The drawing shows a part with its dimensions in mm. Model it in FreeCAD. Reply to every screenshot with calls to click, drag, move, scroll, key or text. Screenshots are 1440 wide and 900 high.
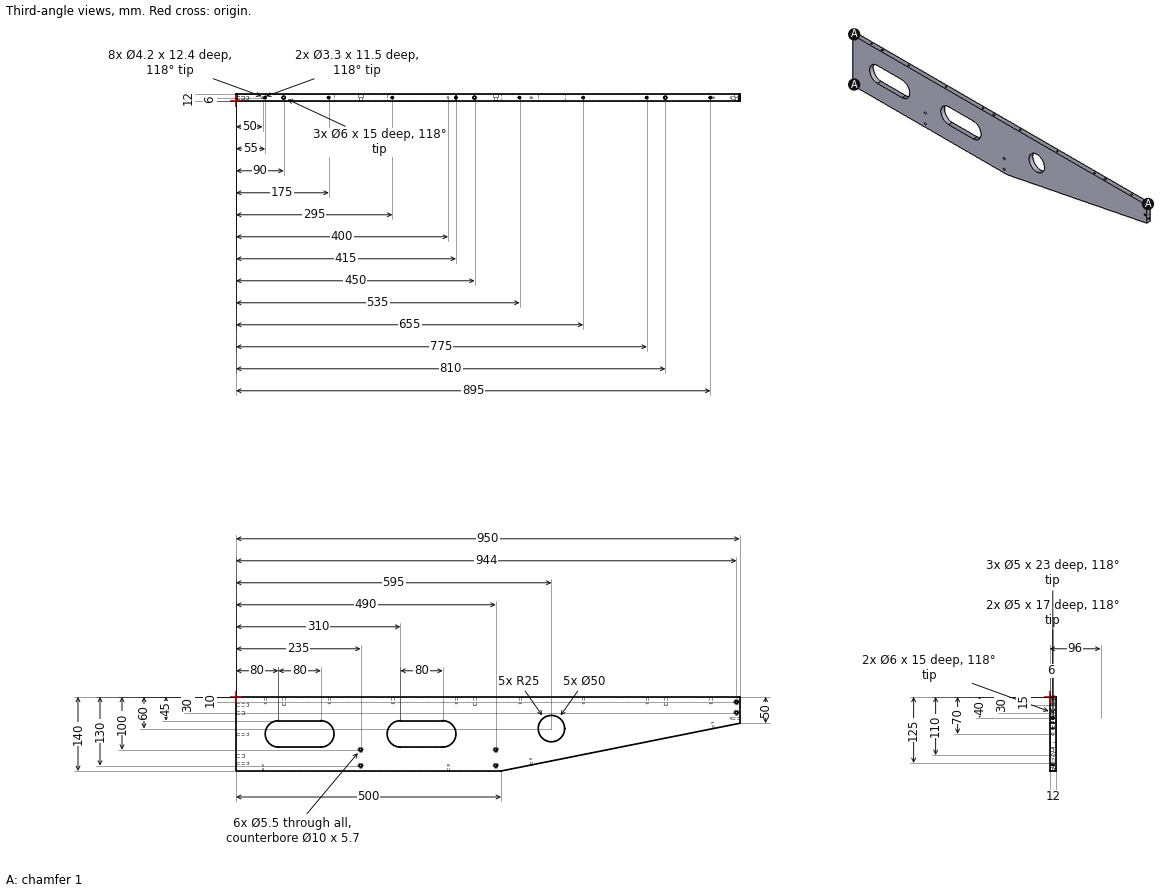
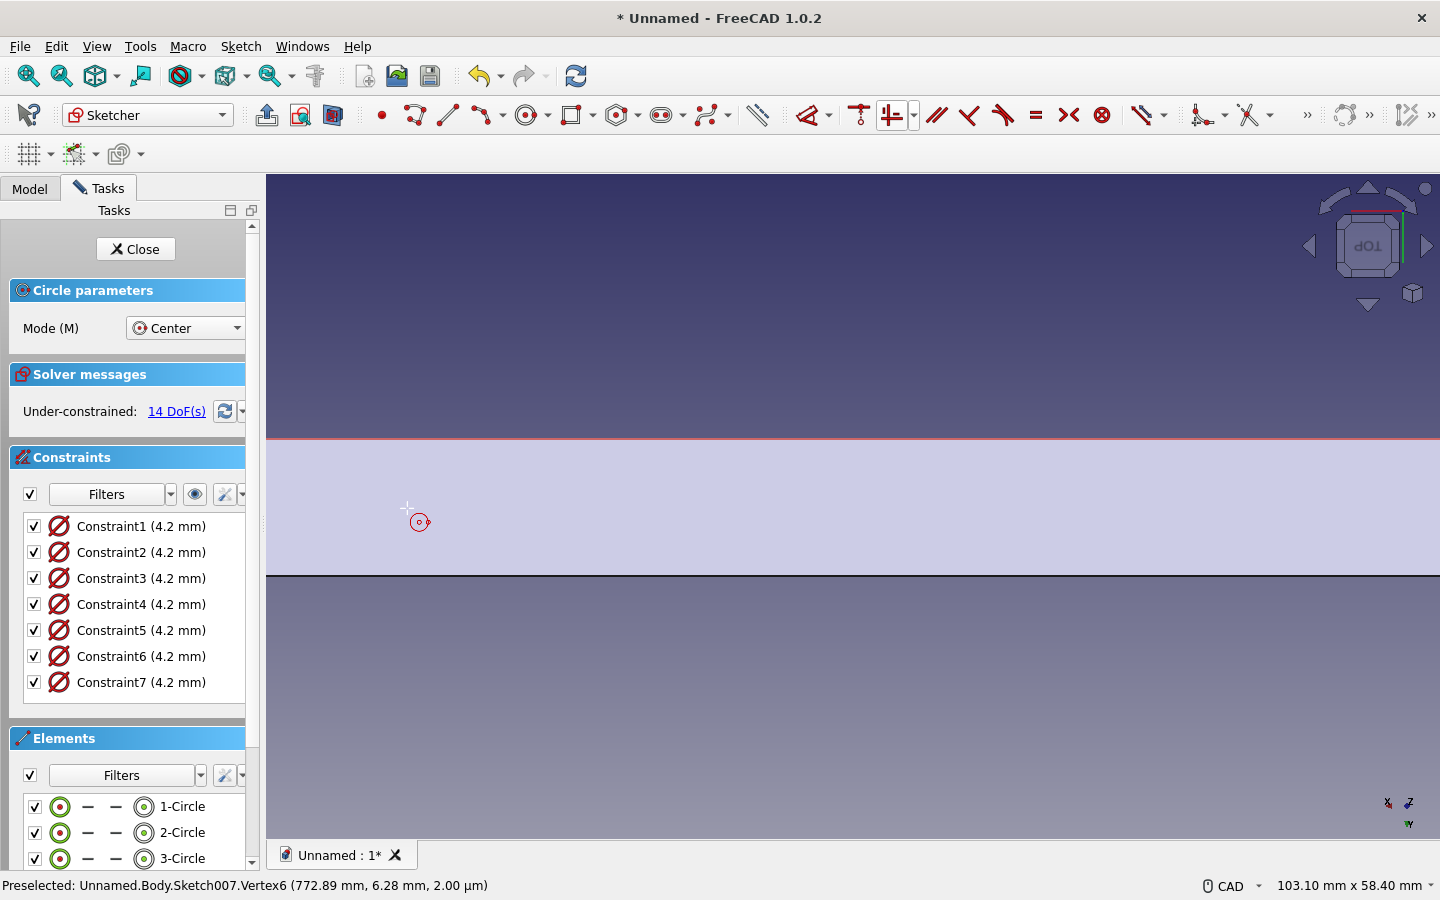
scroll(407, 508, down, 13)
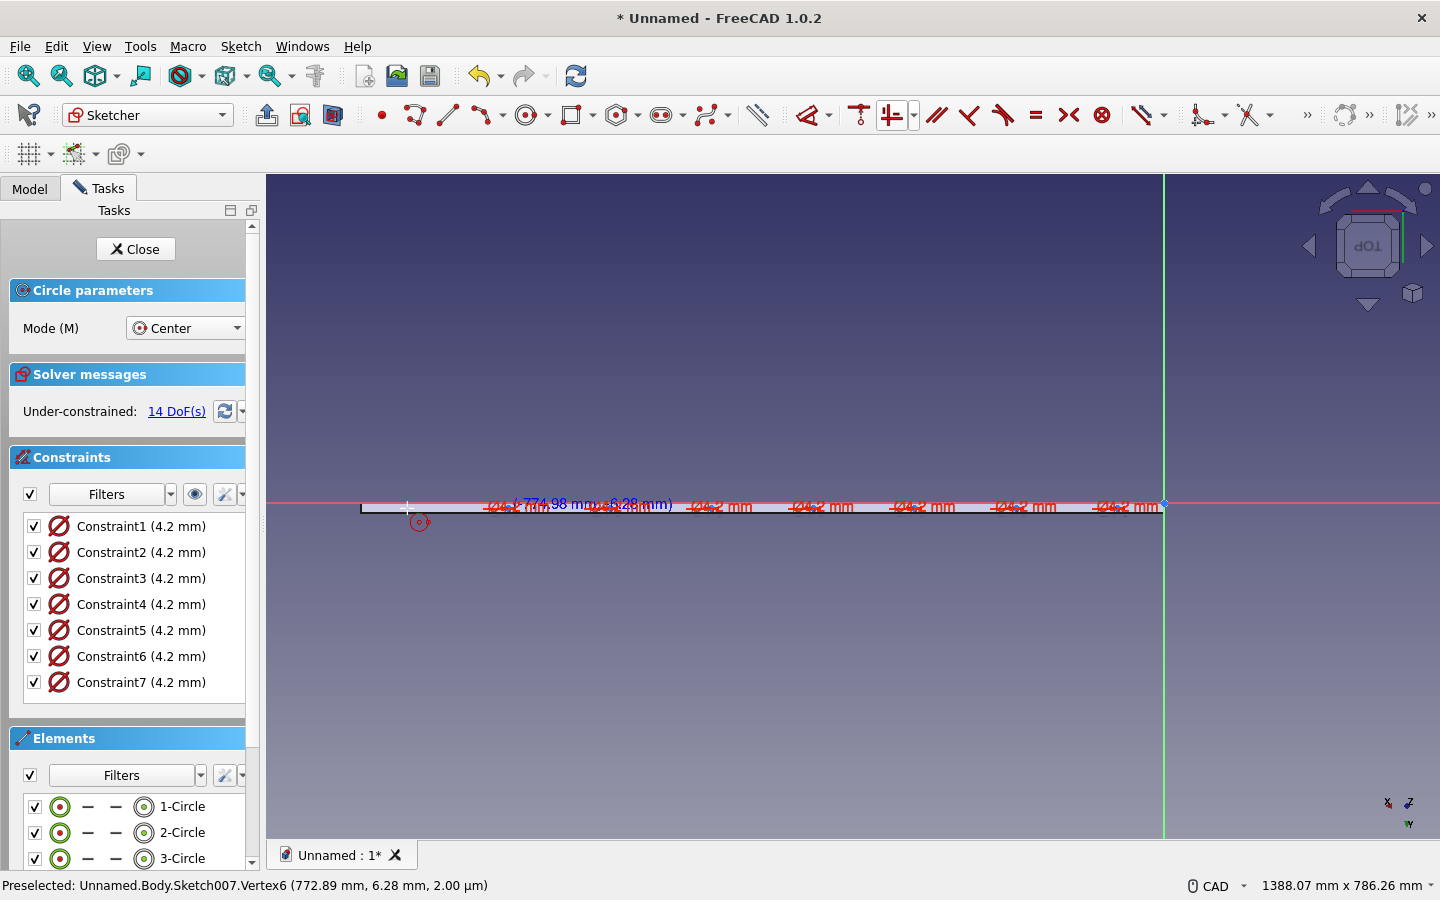
scroll(407, 508, up, 6)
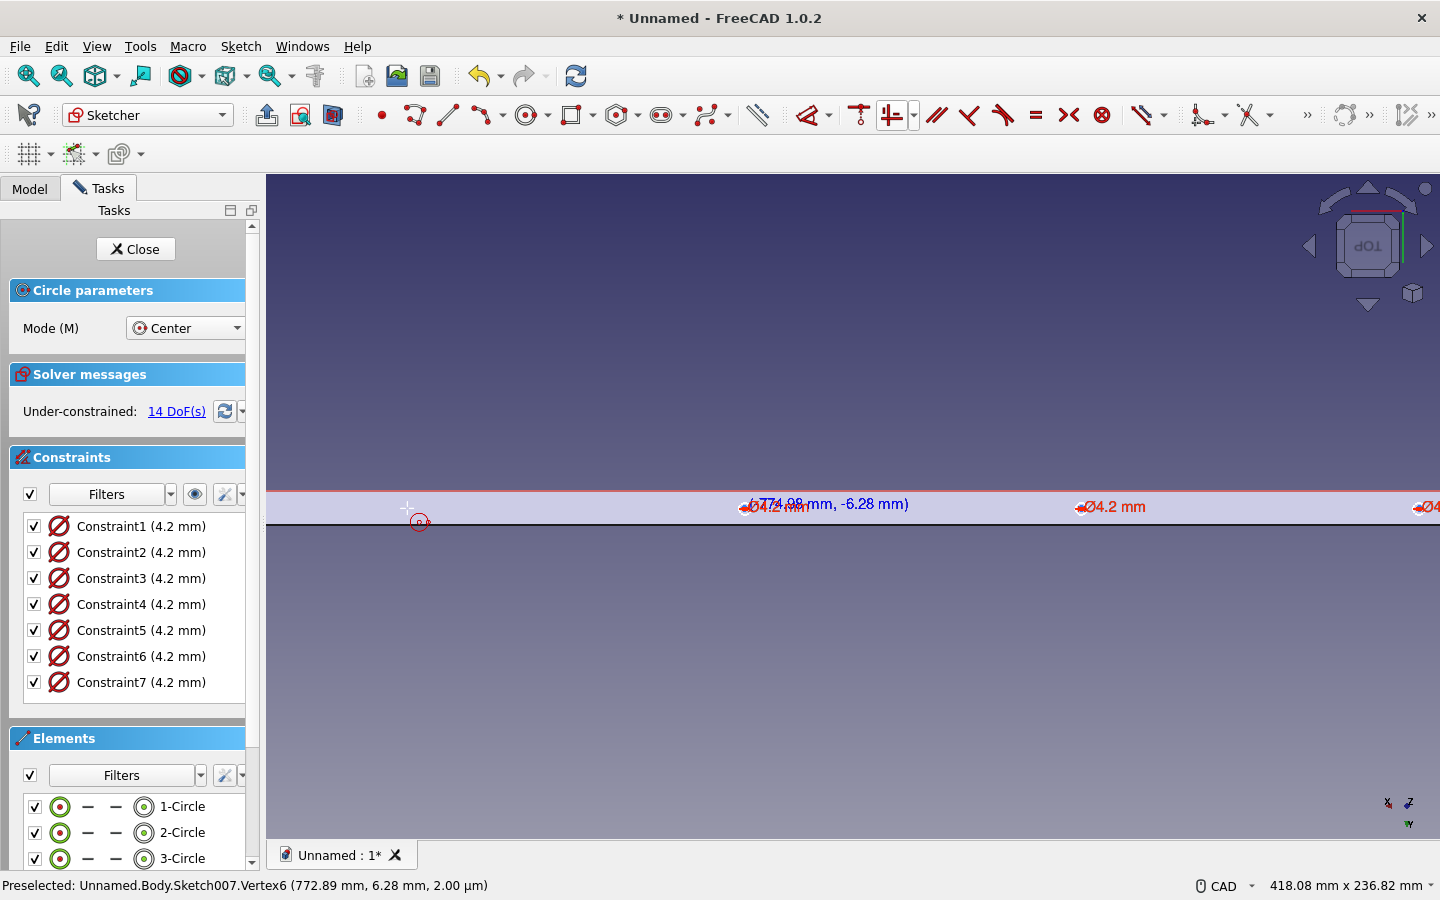
click(408, 508)
move(412, 512)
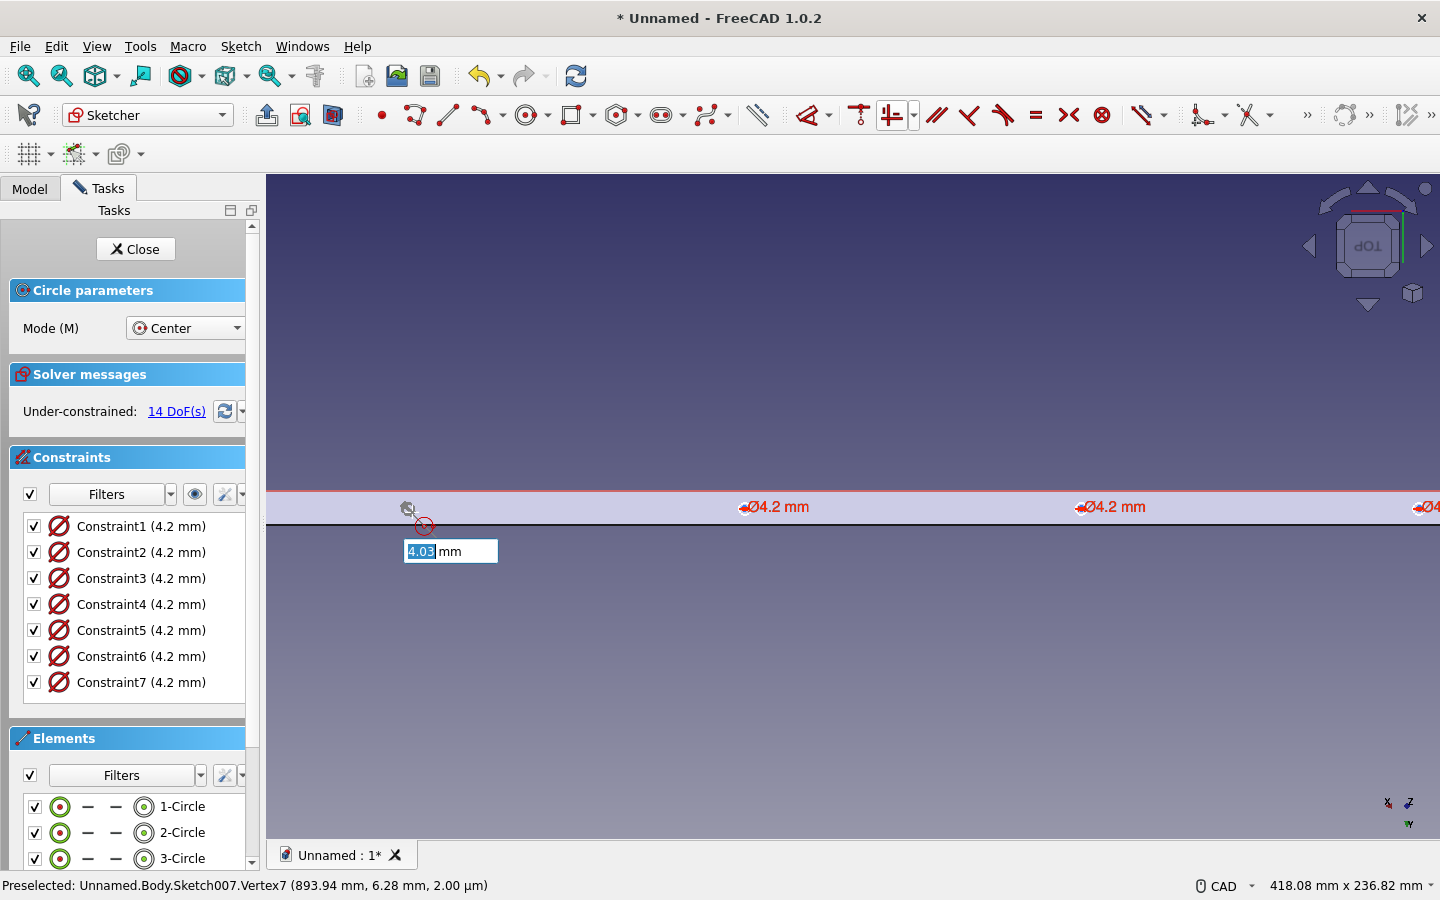
text(4.2)
key(Return)
key(Escape)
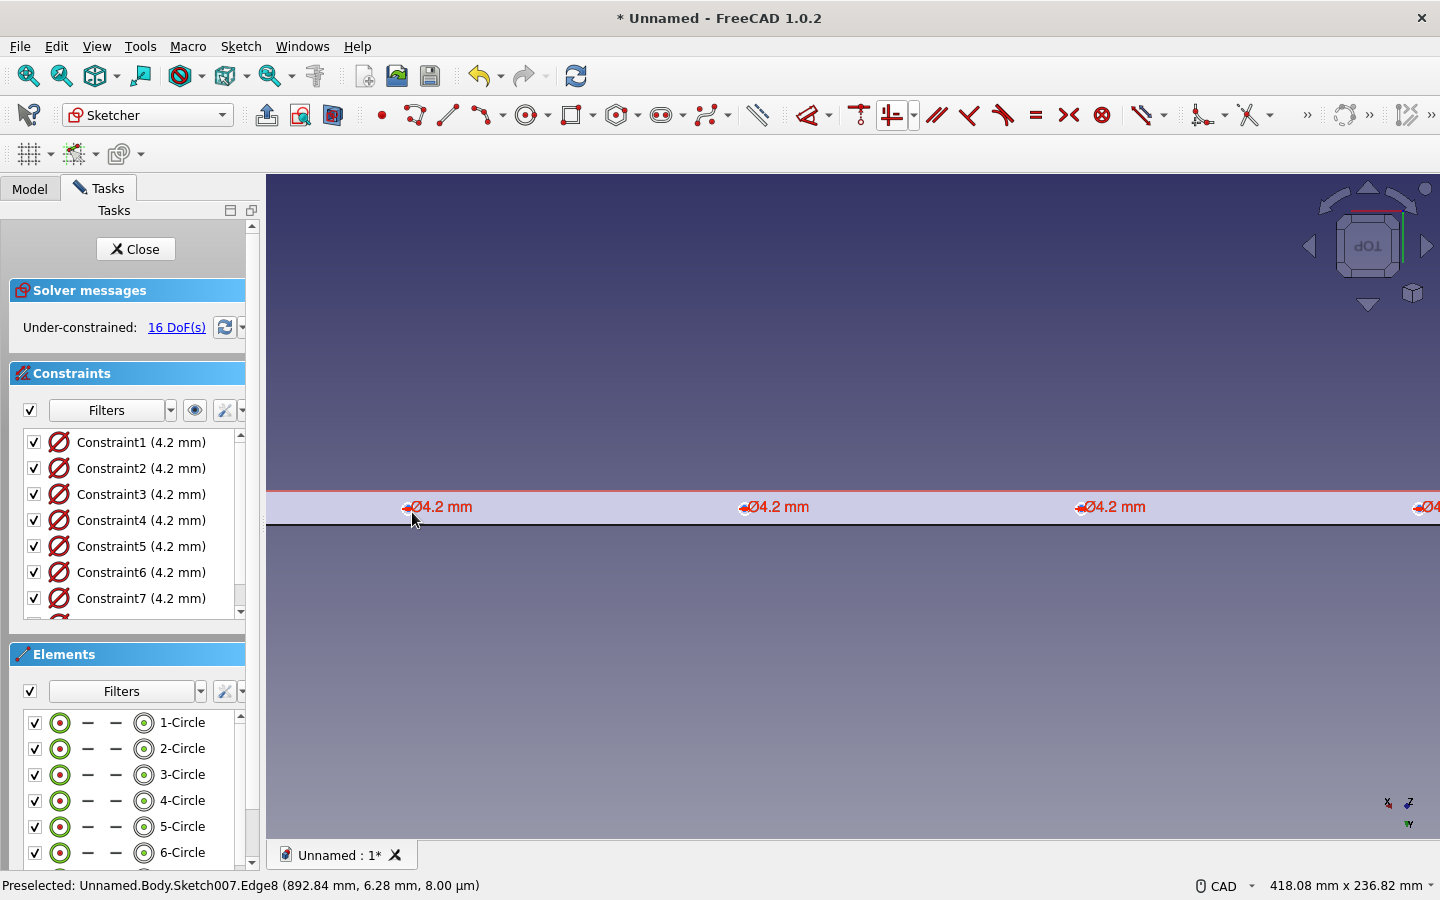
click(806, 116)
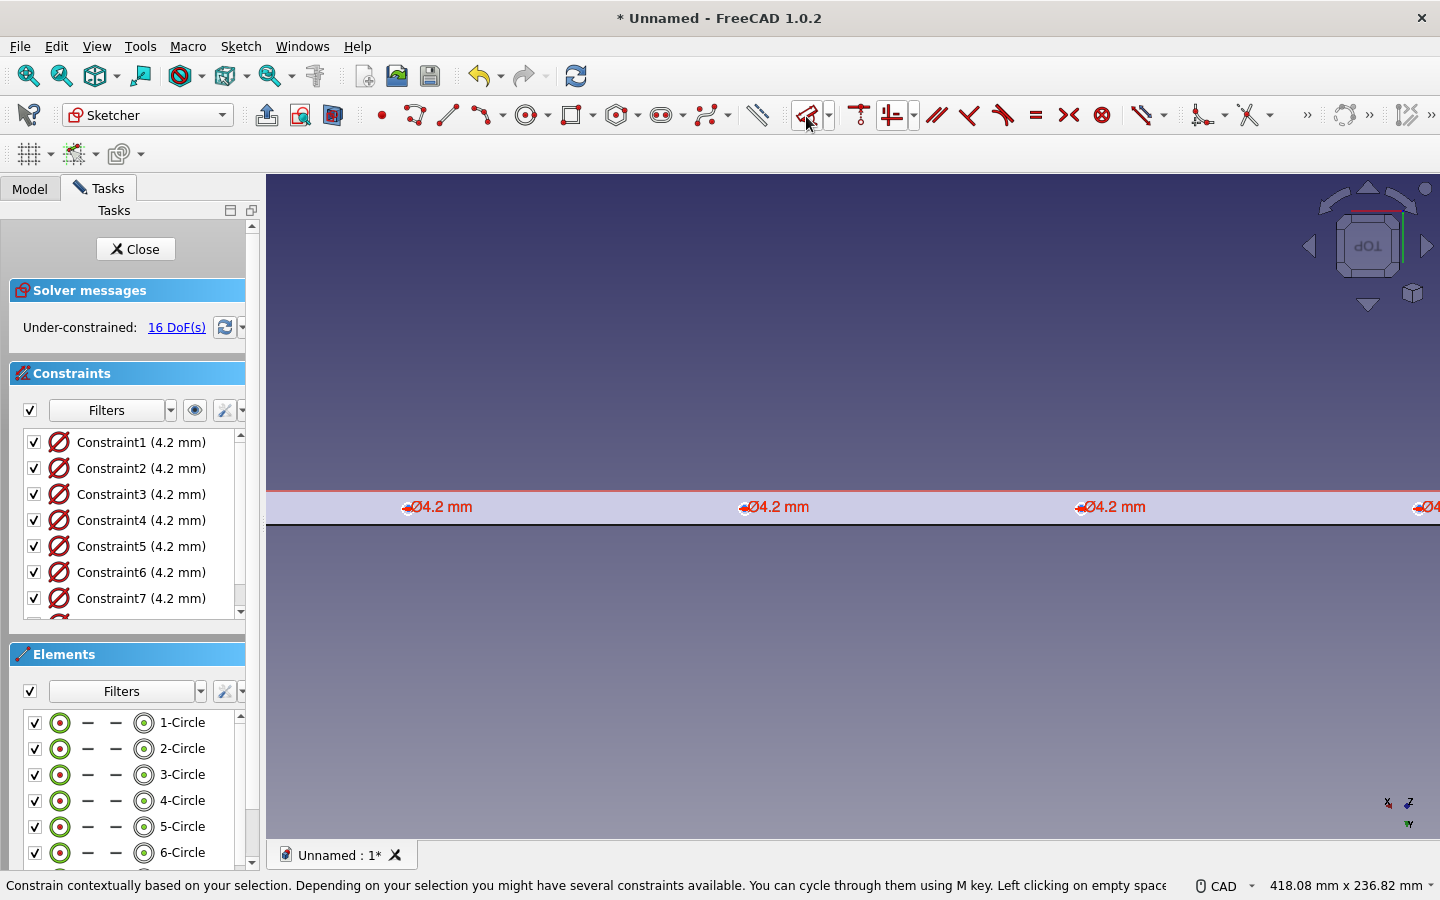
scroll(406, 508, down, 6)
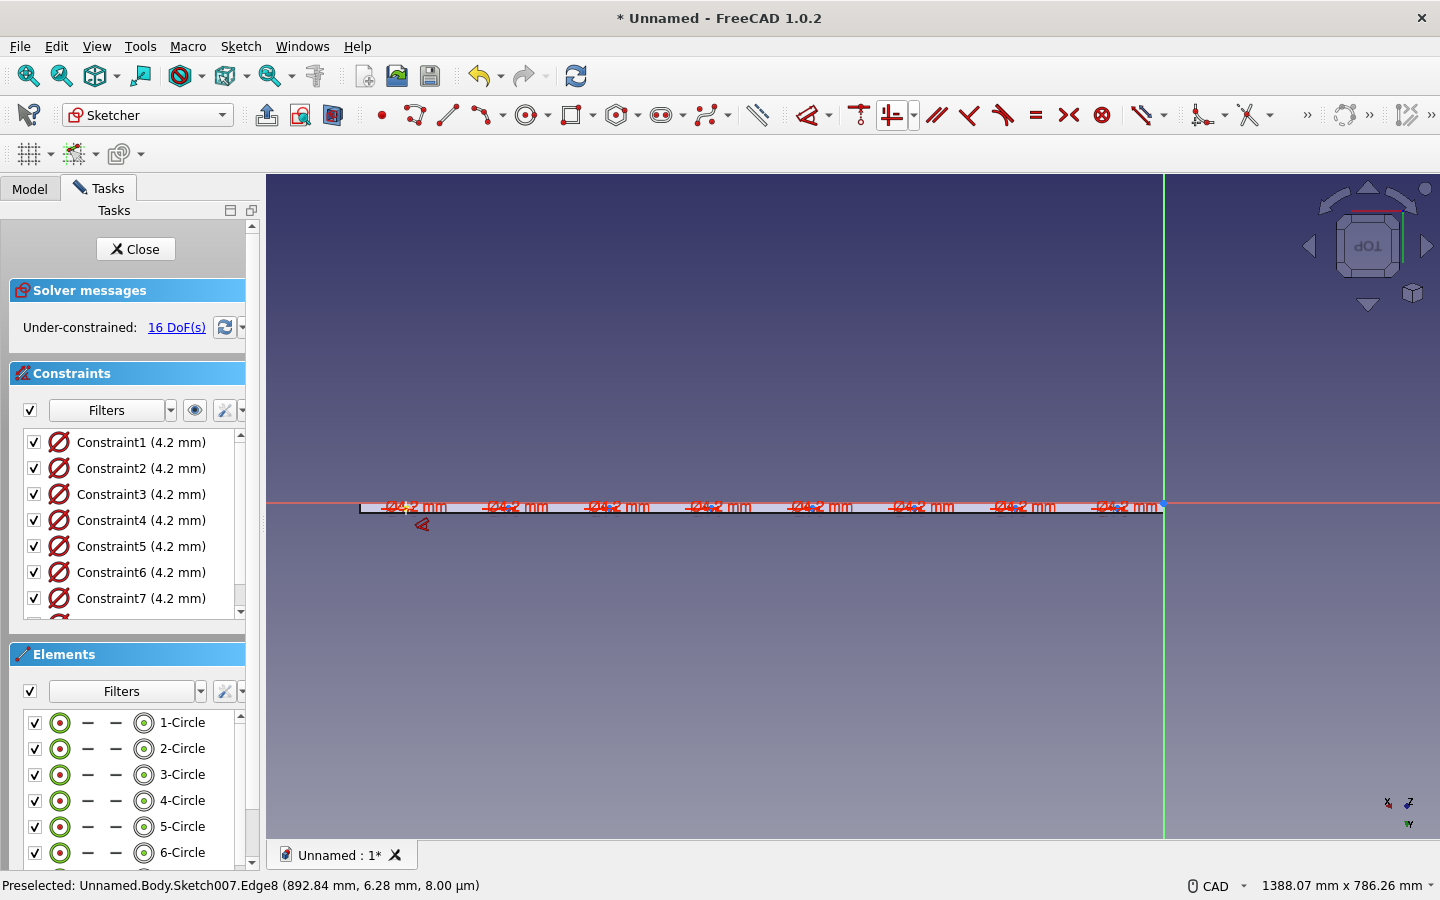
scroll(1117, 509, up, 11)